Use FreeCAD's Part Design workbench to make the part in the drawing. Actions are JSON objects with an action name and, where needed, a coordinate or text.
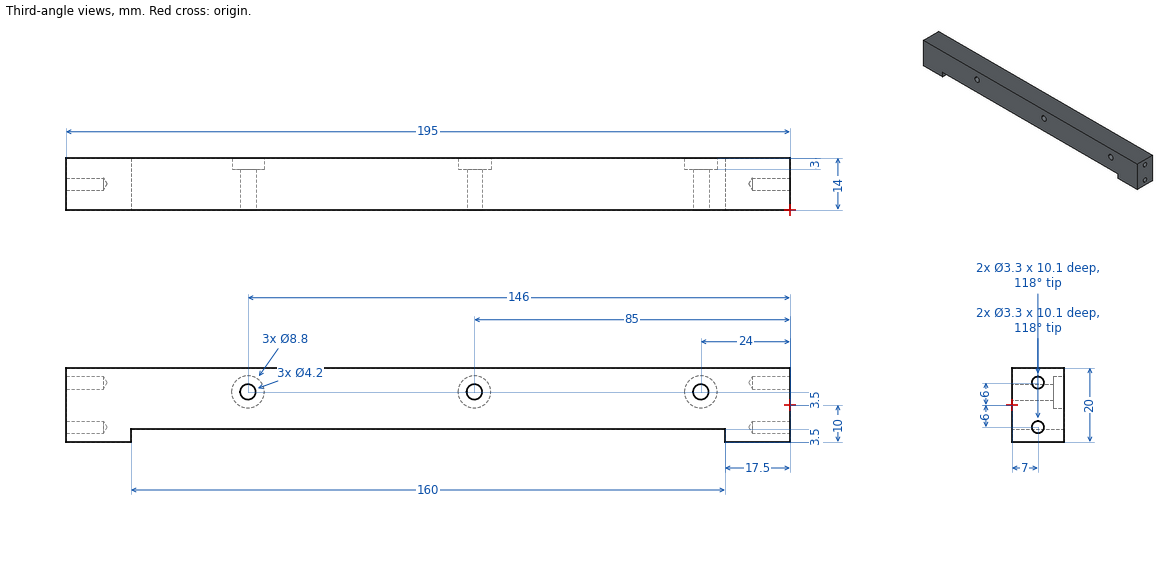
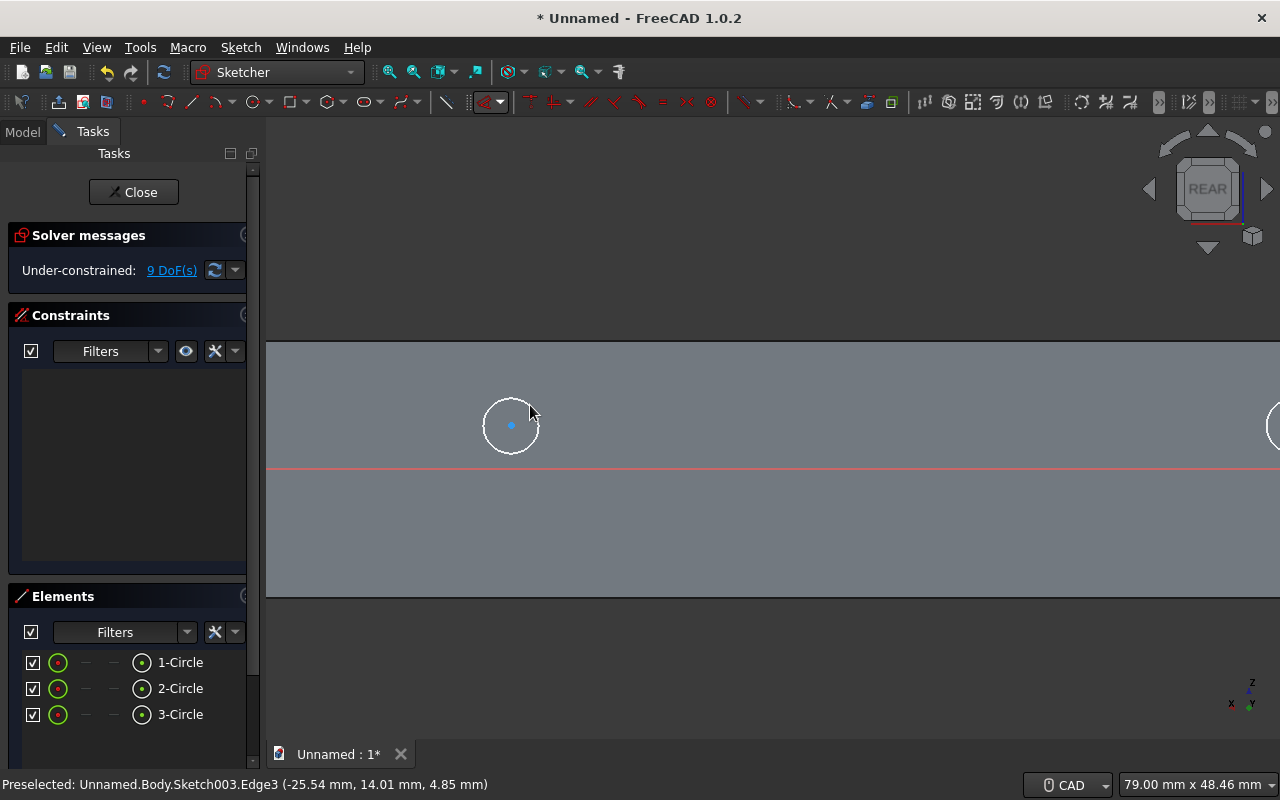
{"action": "scroll", "coordinate": [511, 426], "scroll_direction": "down", "scroll_amount": 6}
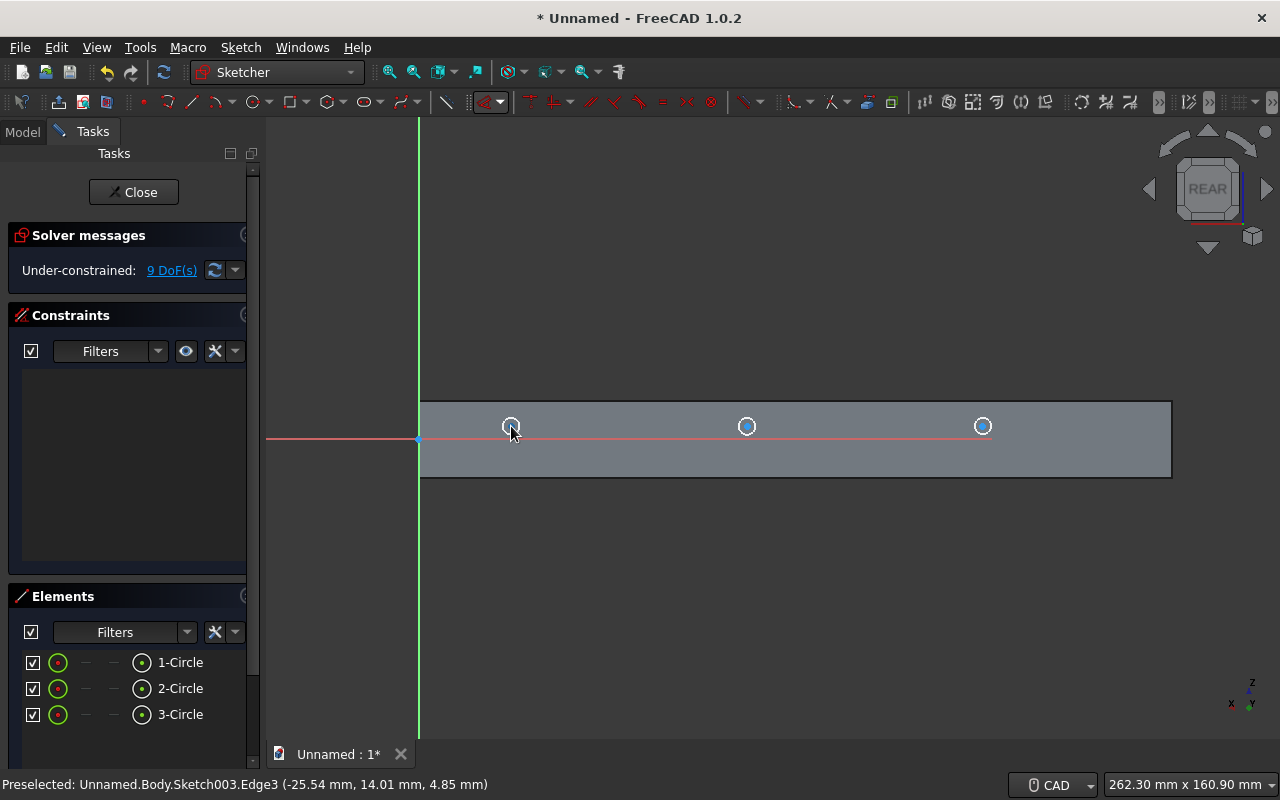
{"action": "scroll", "coordinate": [989, 420], "scroll_direction": "up", "scroll_amount": 3}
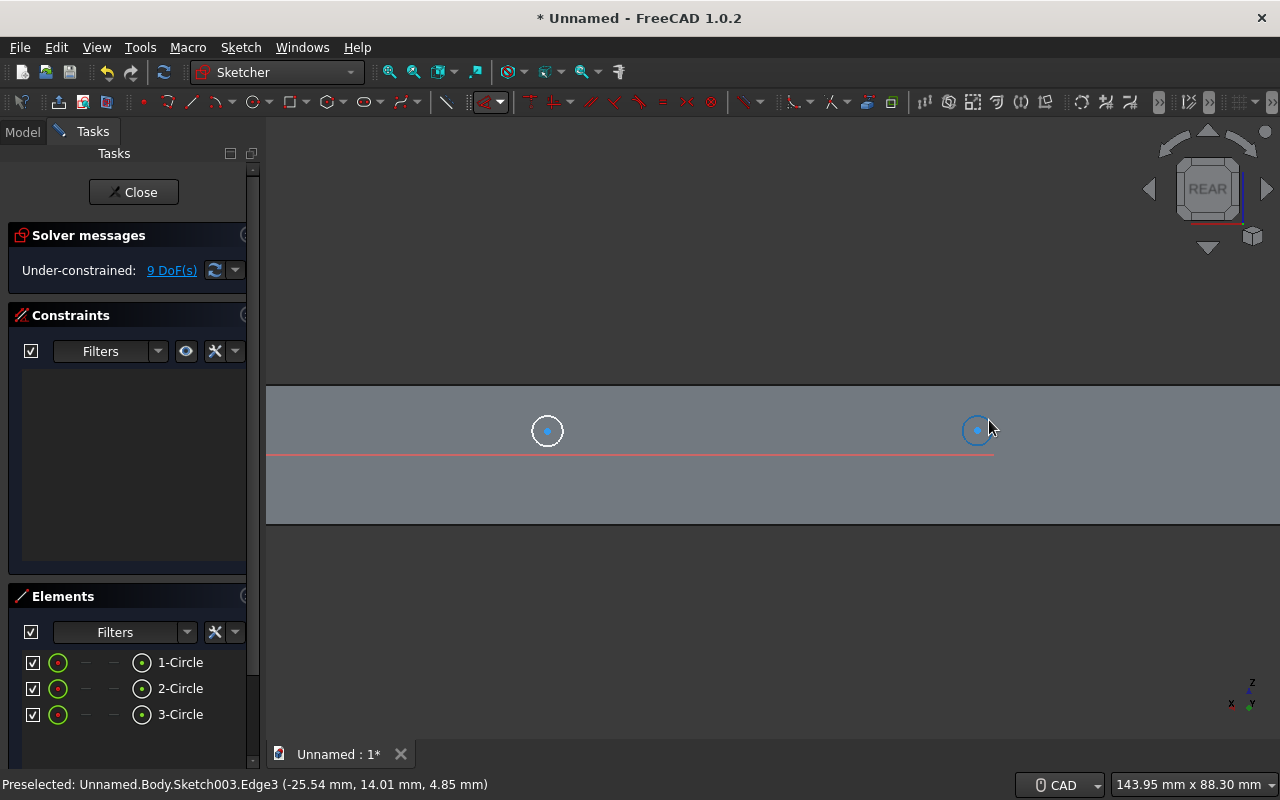
{"action": "left_click", "coordinate": [988, 420]}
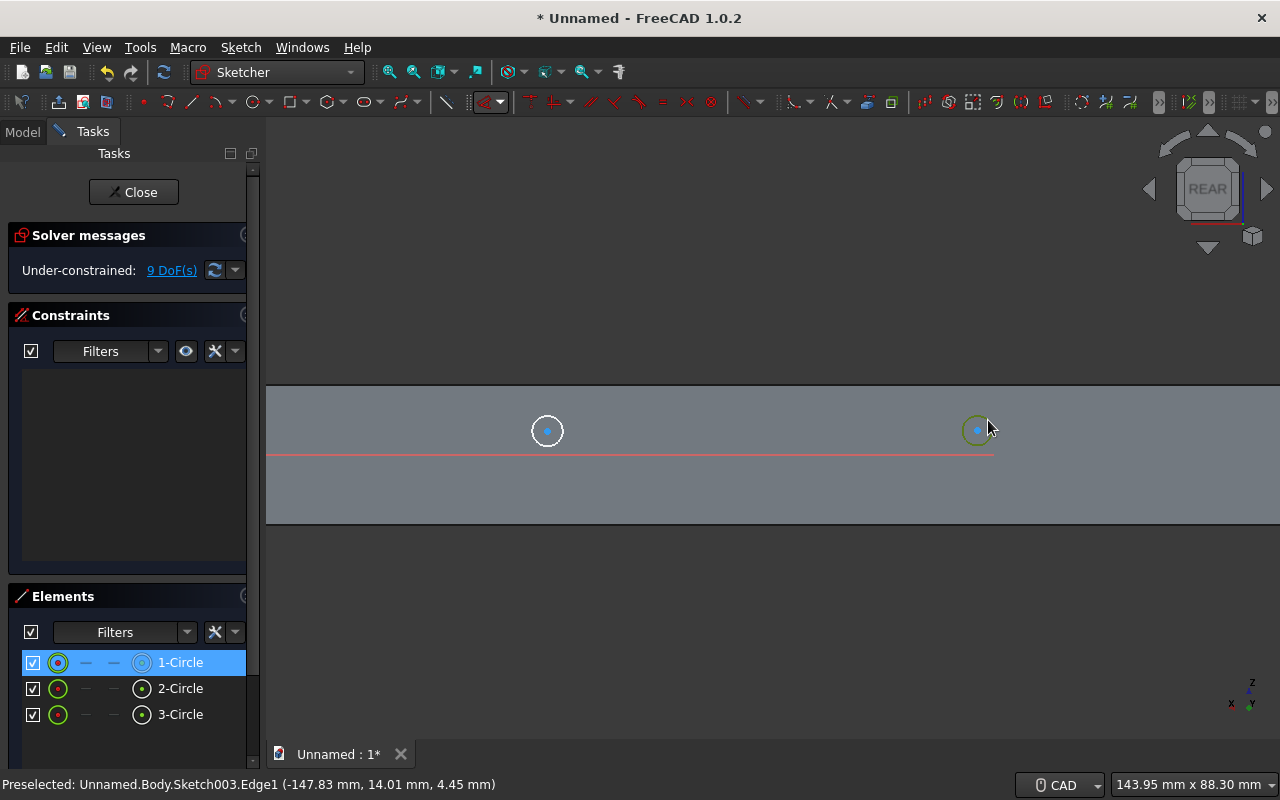
{"action": "left_click", "coordinate": [558, 420]}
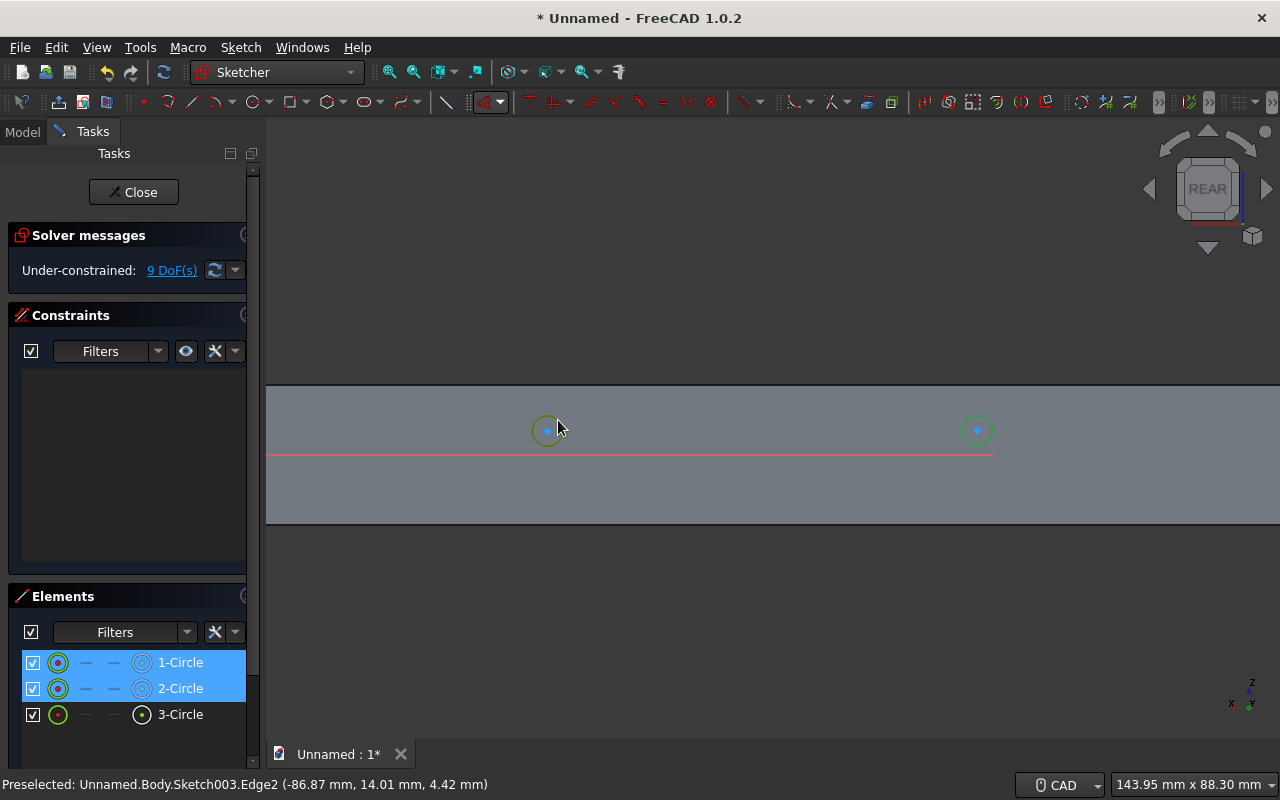
{"action": "scroll", "coordinate": [989, 419], "scroll_direction": "down", "scroll_amount": 3}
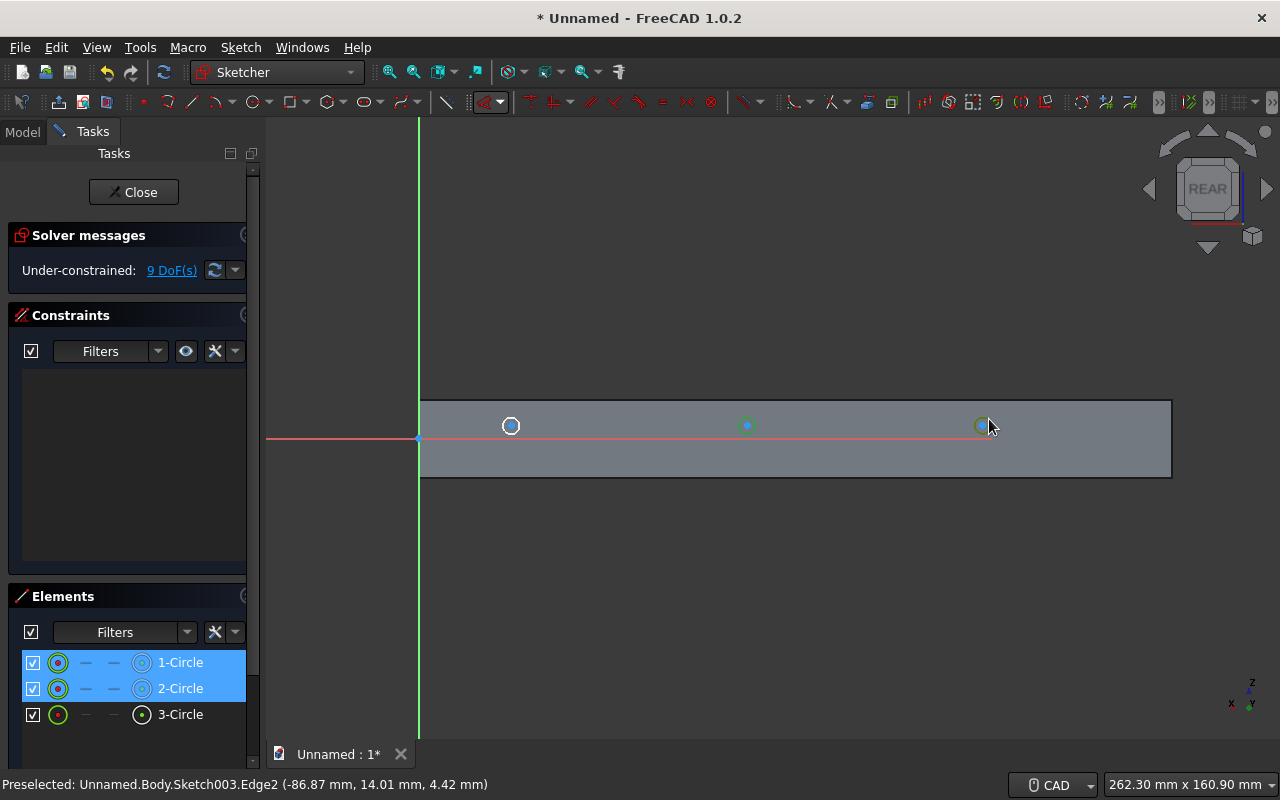
{"action": "scroll", "coordinate": [517, 420], "scroll_direction": "up", "scroll_amount": 3}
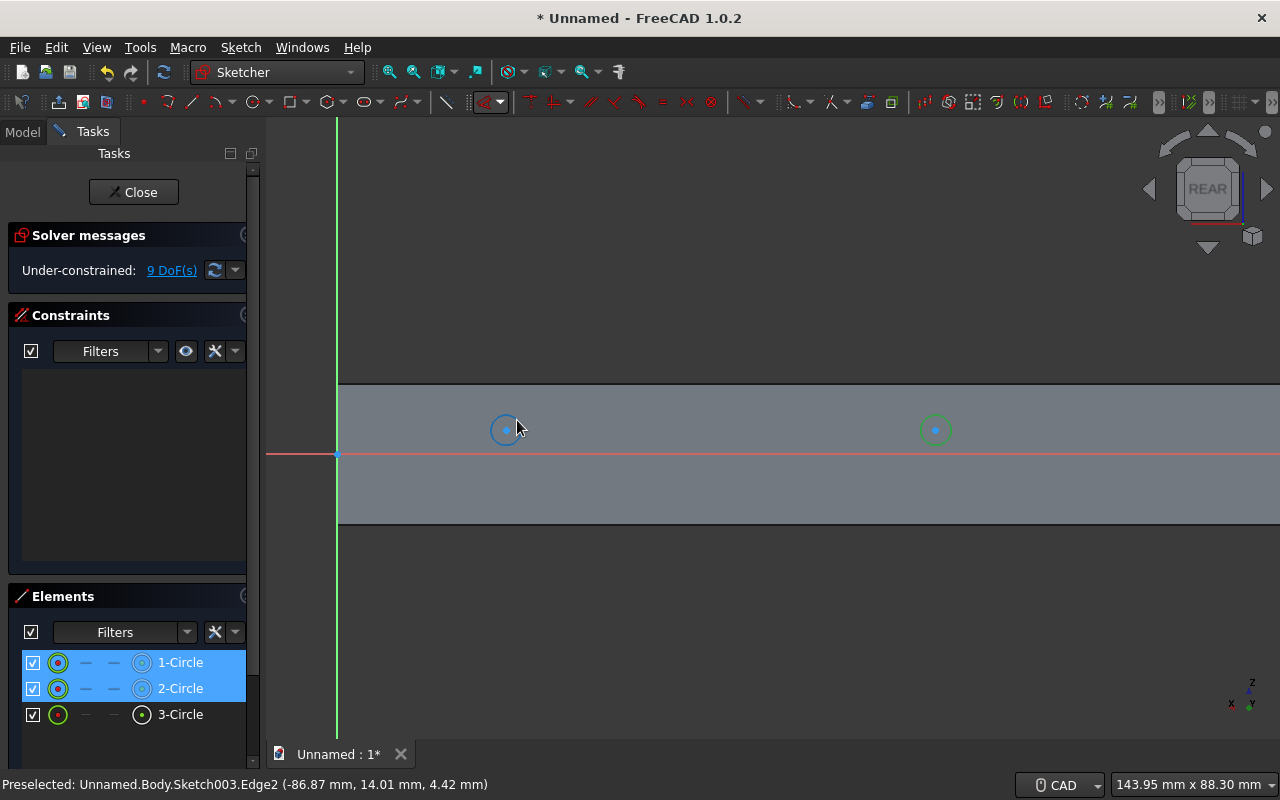
{"action": "left_click", "coordinate": [517, 420]}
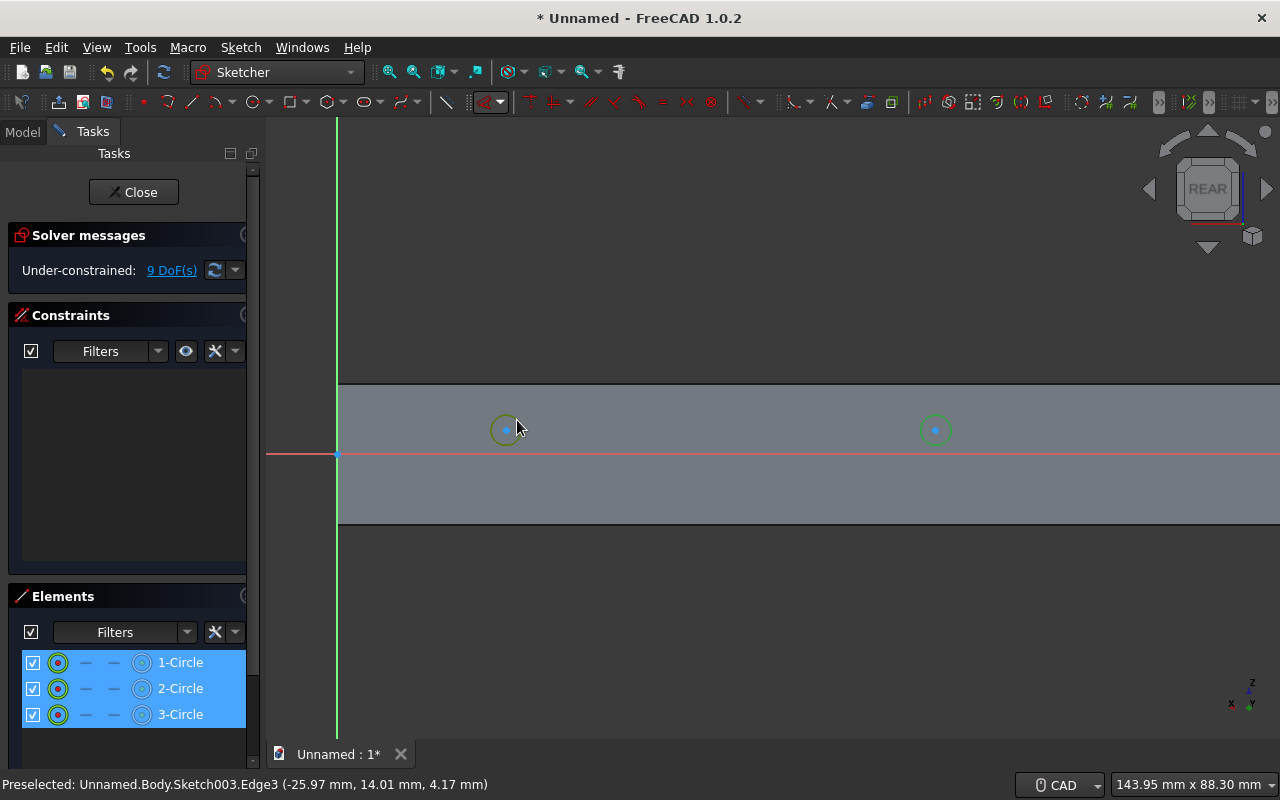
{"action": "left_click", "coordinate": [664, 102]}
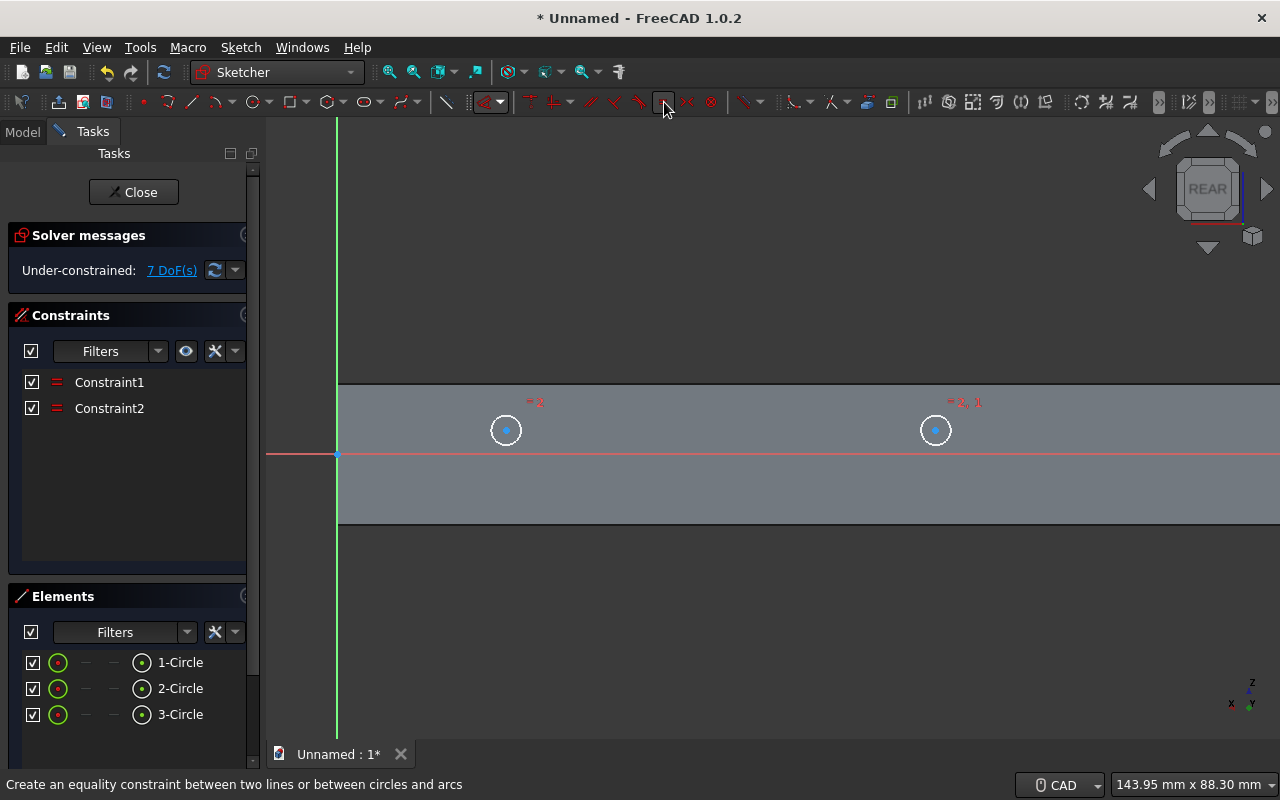
{"action": "scroll", "coordinate": [517, 420], "scroll_direction": "down", "scroll_amount": 3}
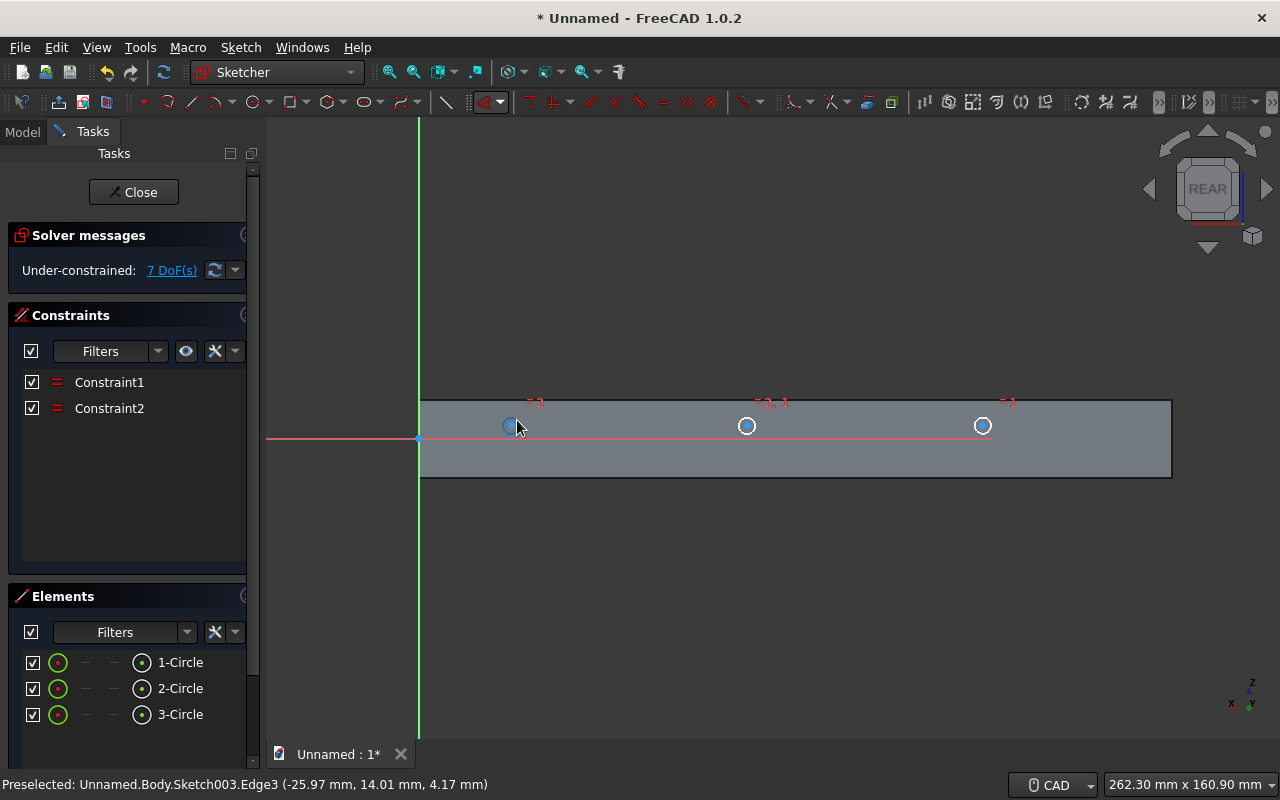
{"action": "scroll", "coordinate": [989, 420], "scroll_direction": "up", "scroll_amount": 5}